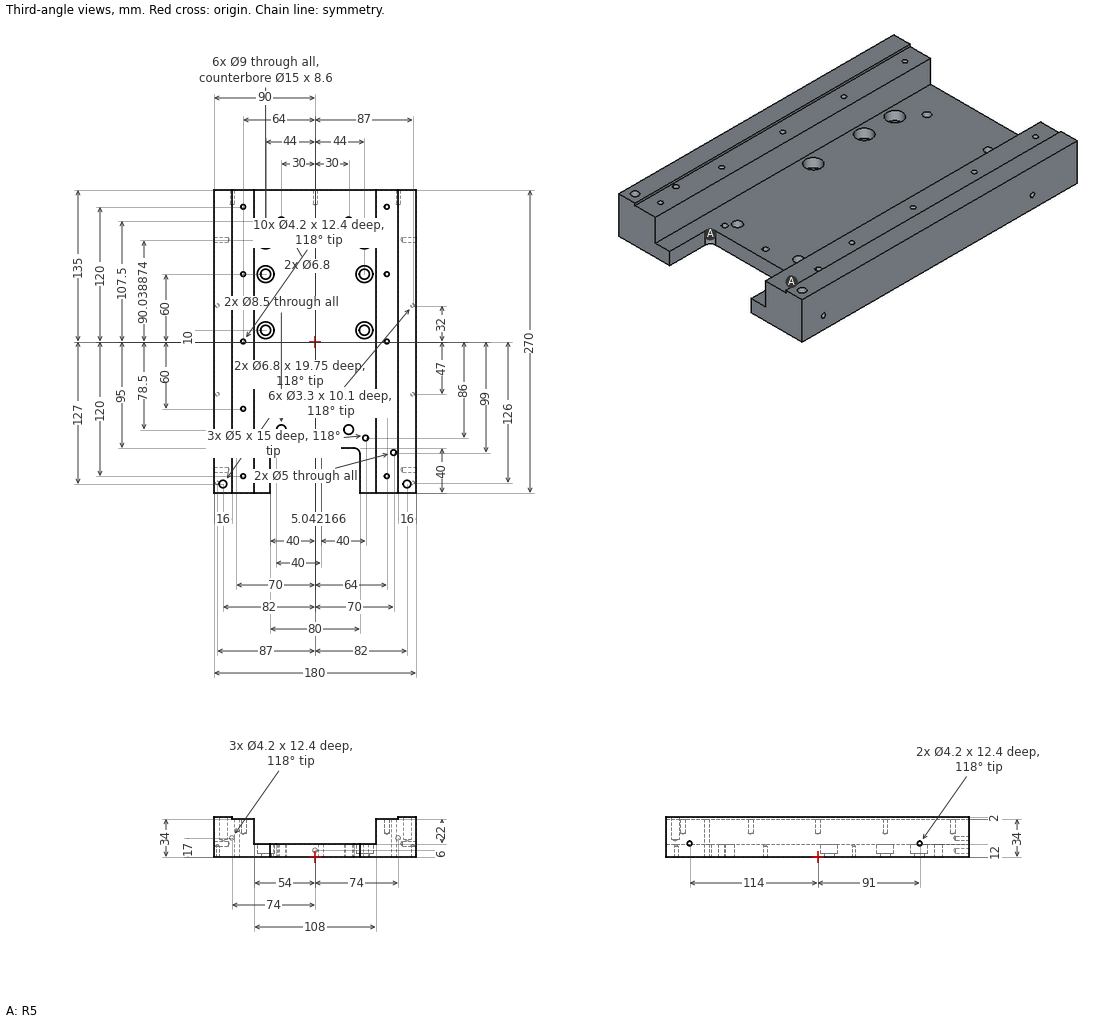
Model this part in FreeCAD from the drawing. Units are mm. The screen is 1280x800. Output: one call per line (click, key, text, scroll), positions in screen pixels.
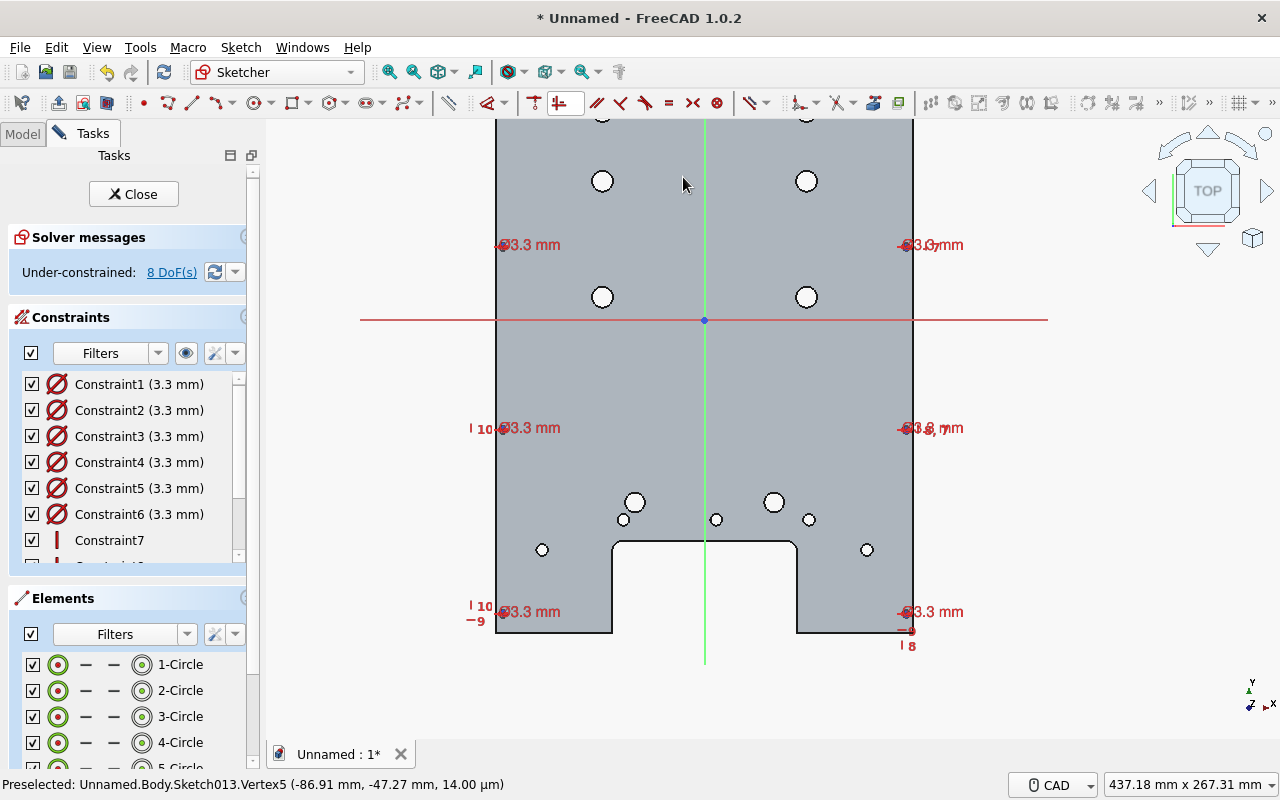
click(906, 430)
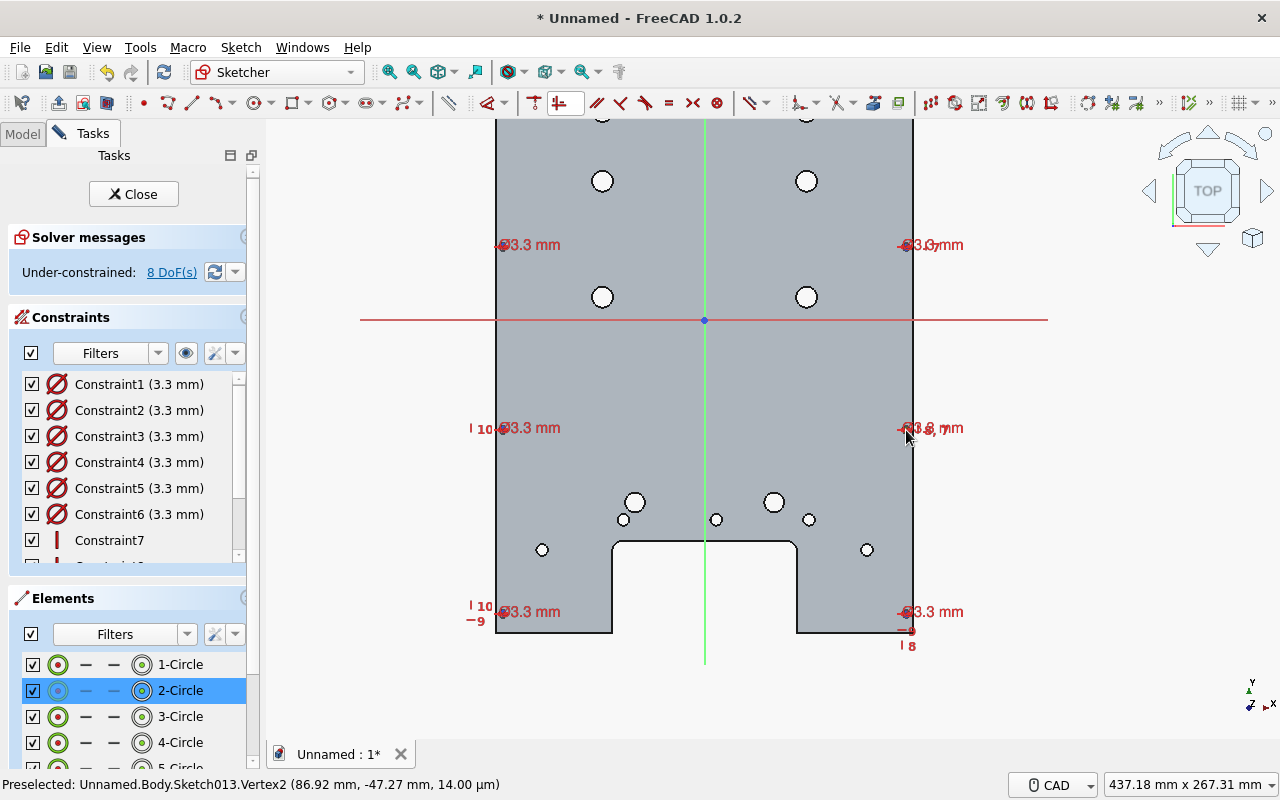
click(503, 430)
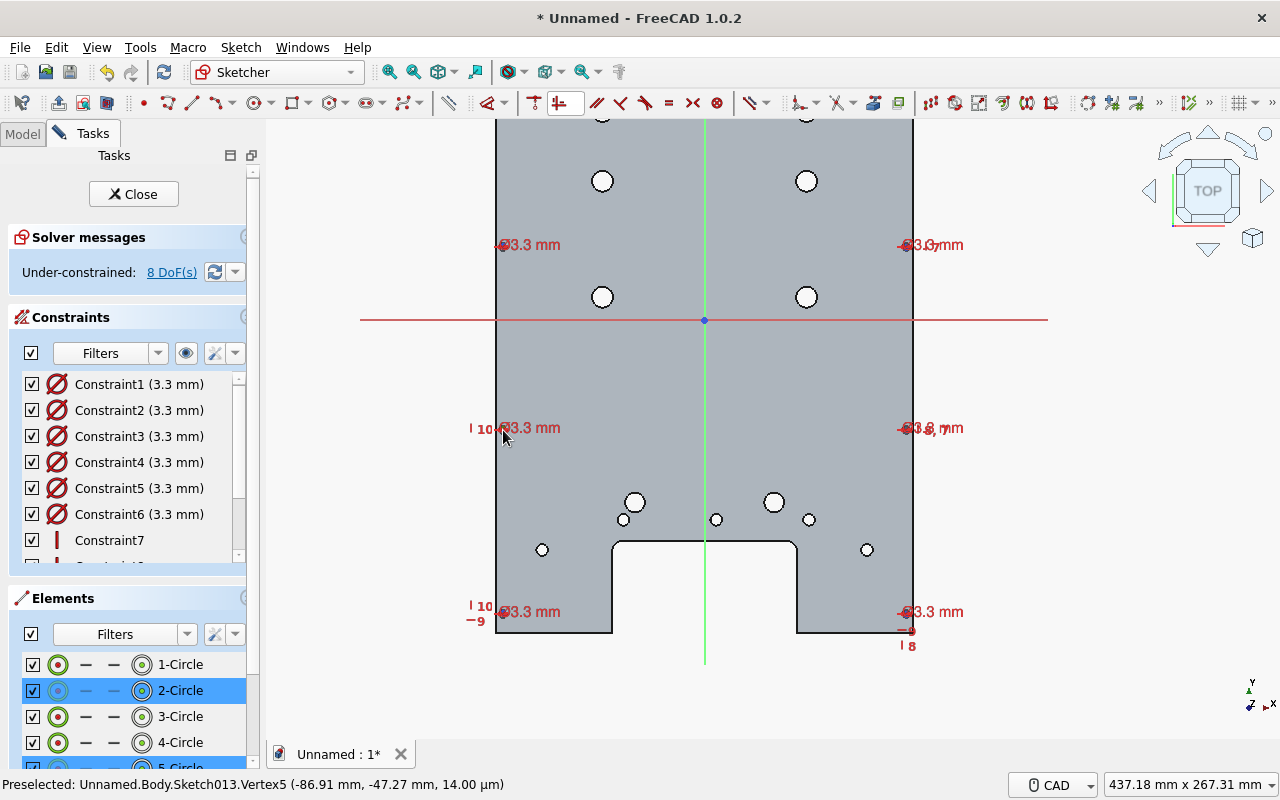
click(578, 104)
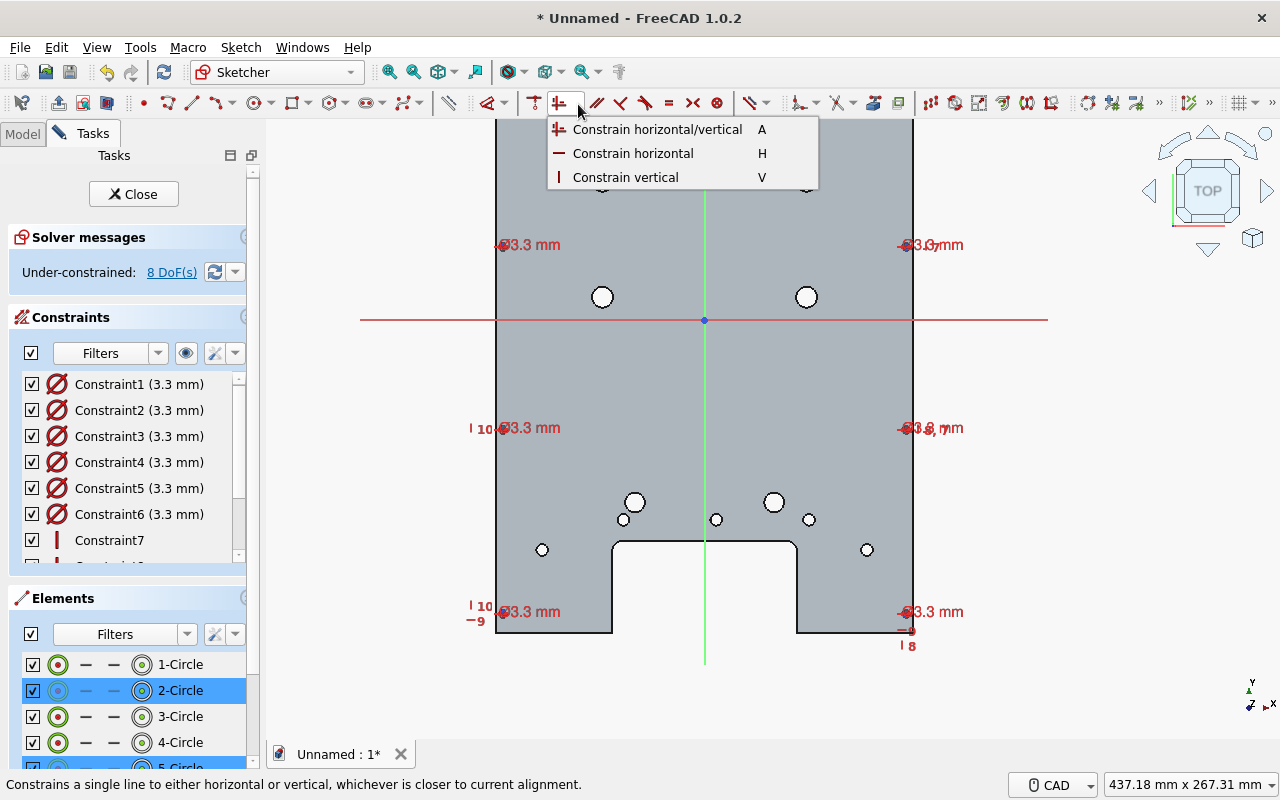
click(683, 153)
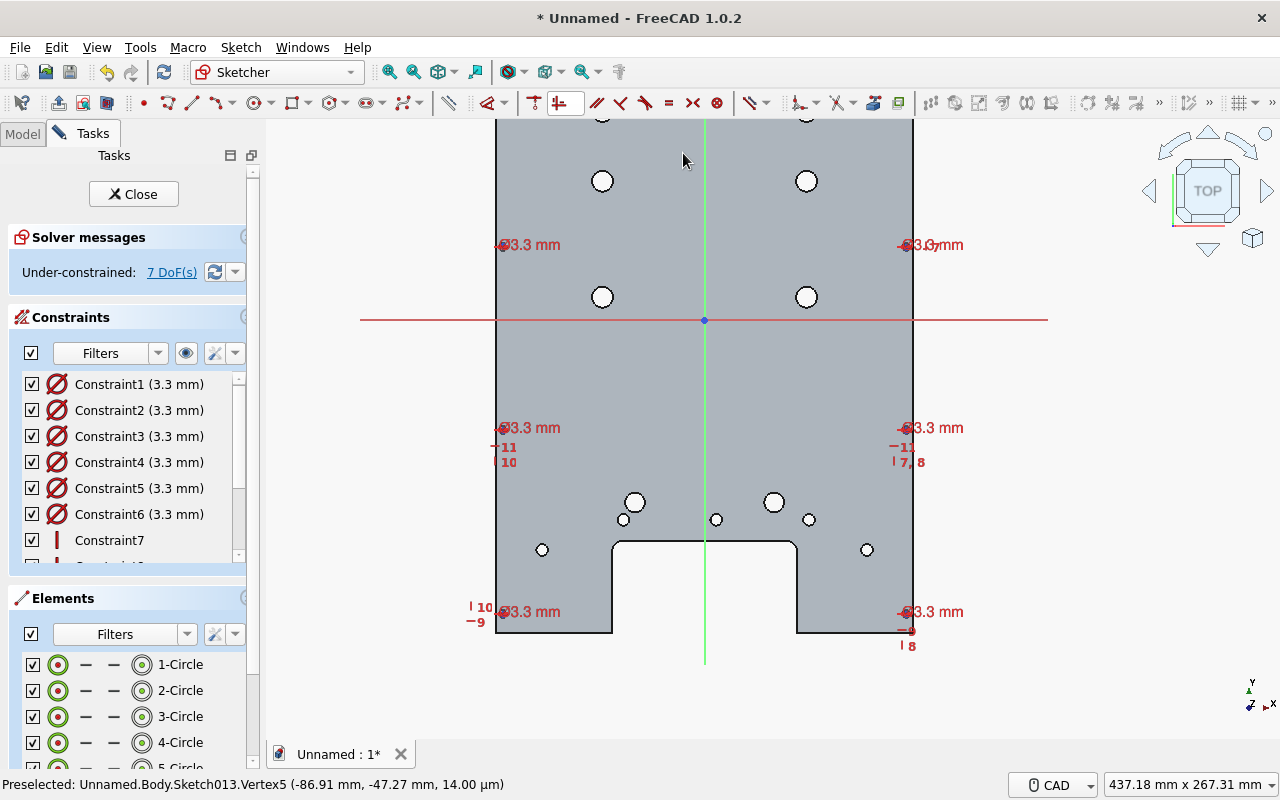
click(503, 430)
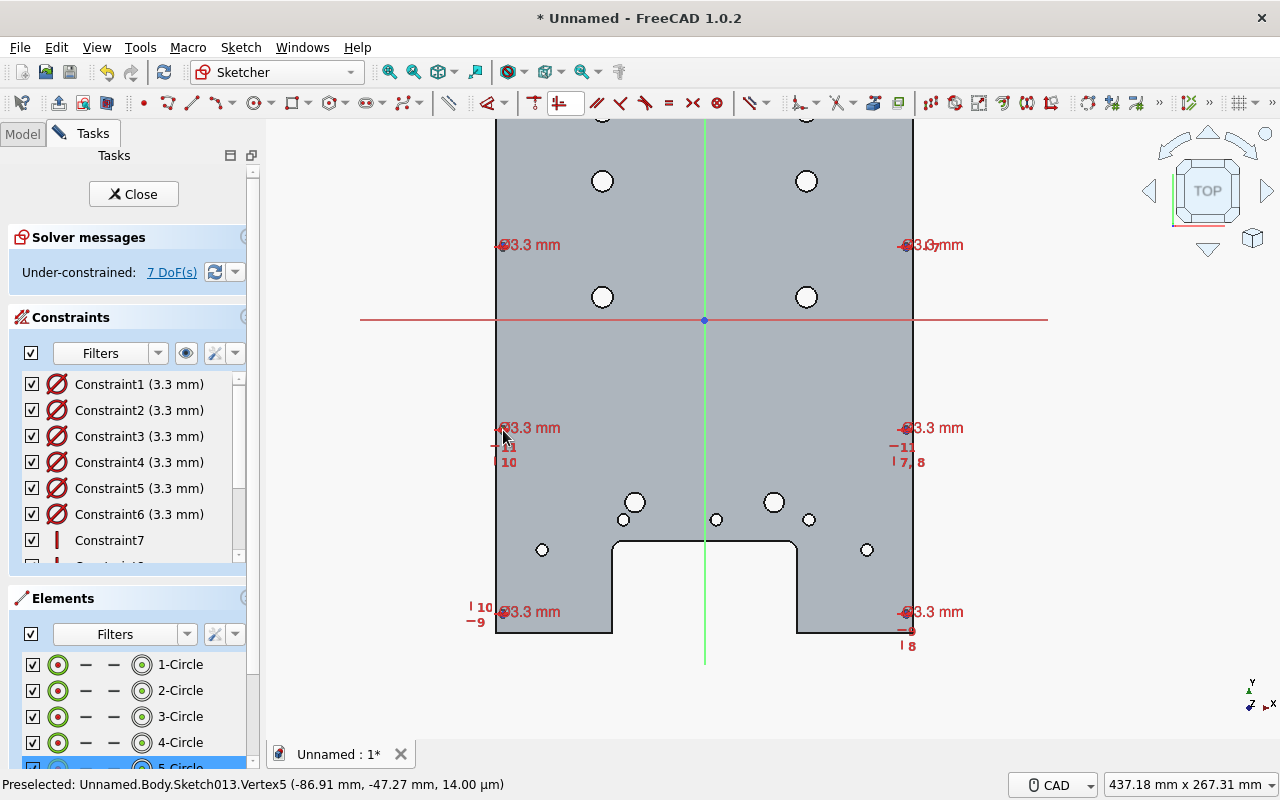
click(503, 247)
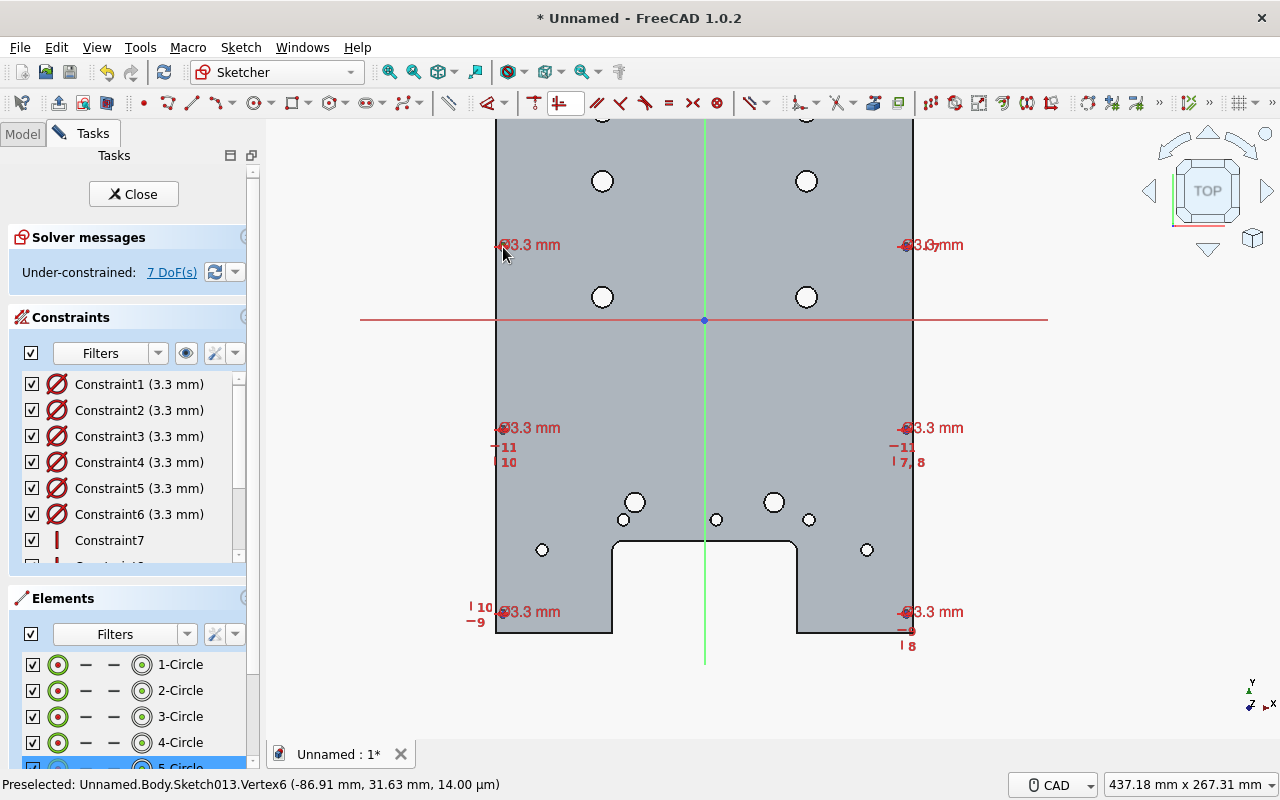
key(v)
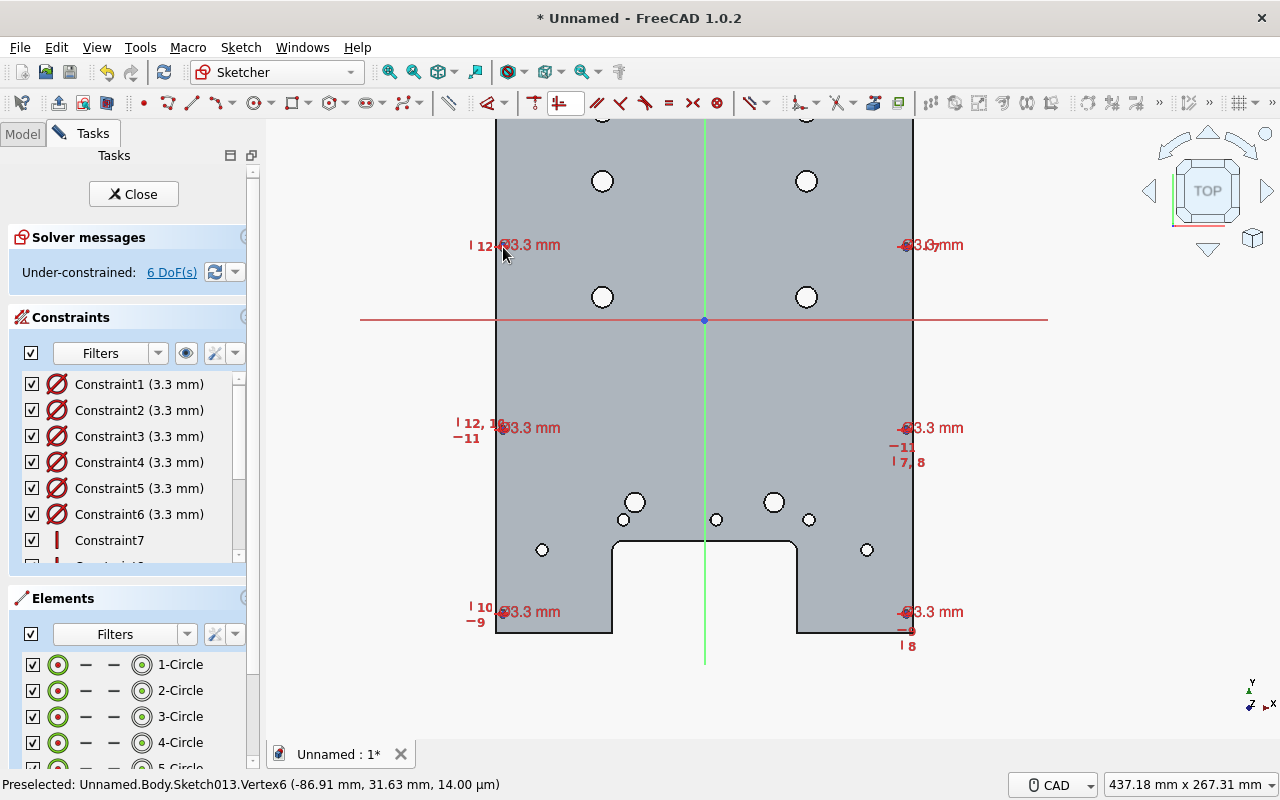
click(906, 247)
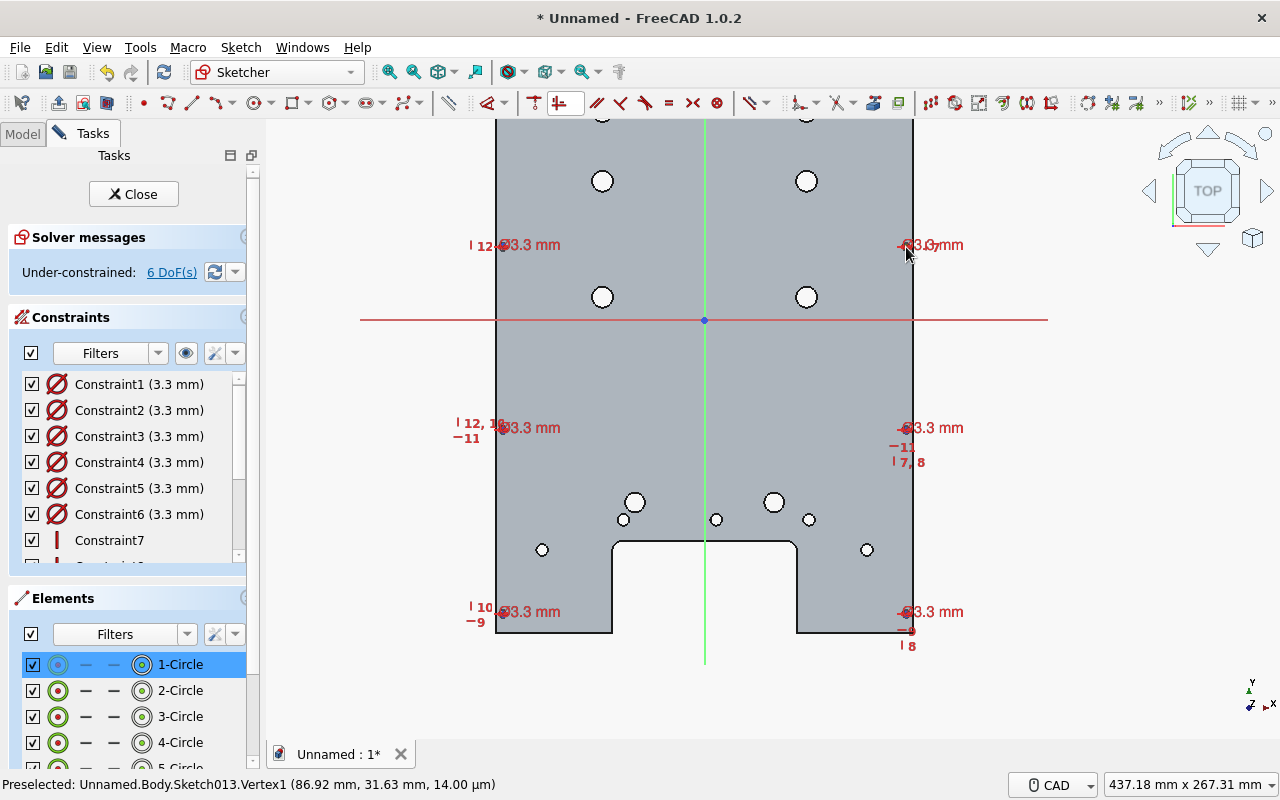
click(503, 247)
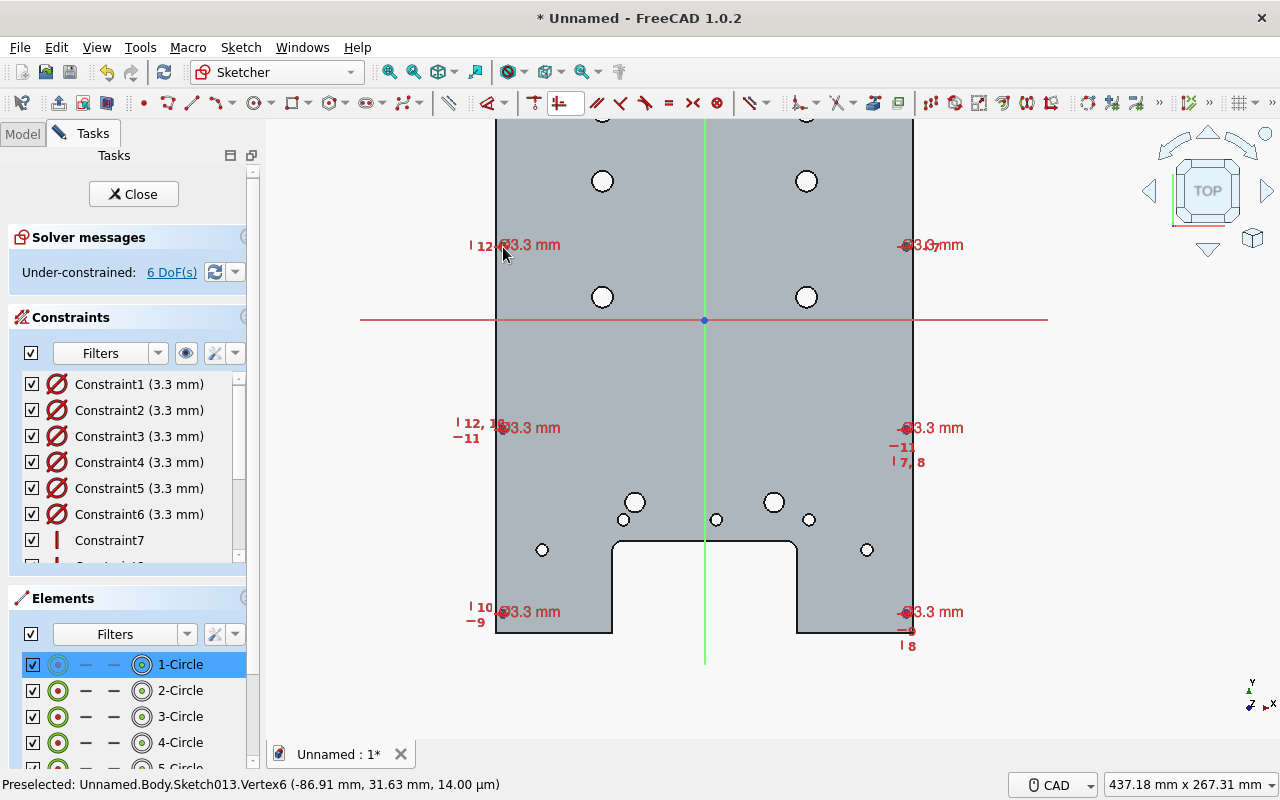
click(578, 104)